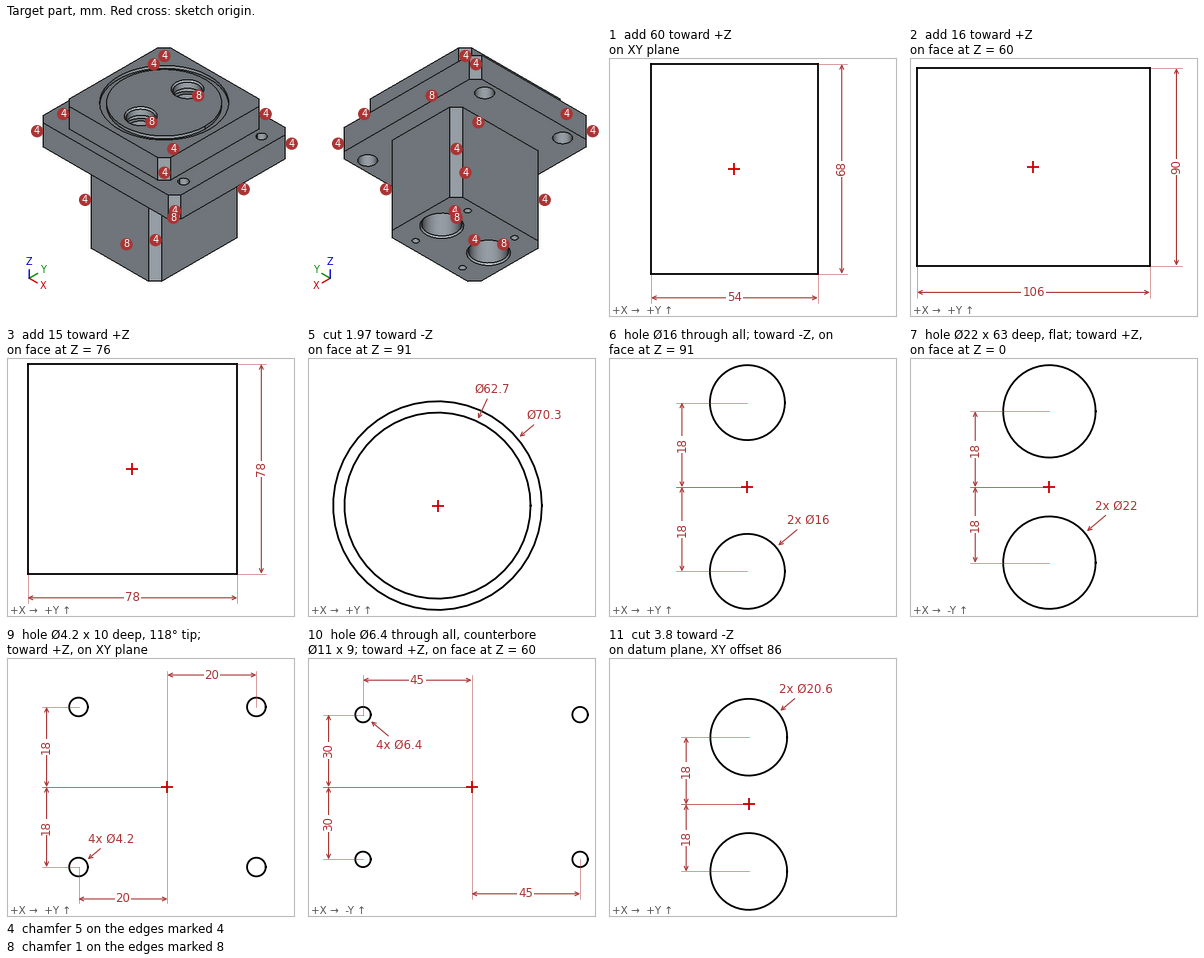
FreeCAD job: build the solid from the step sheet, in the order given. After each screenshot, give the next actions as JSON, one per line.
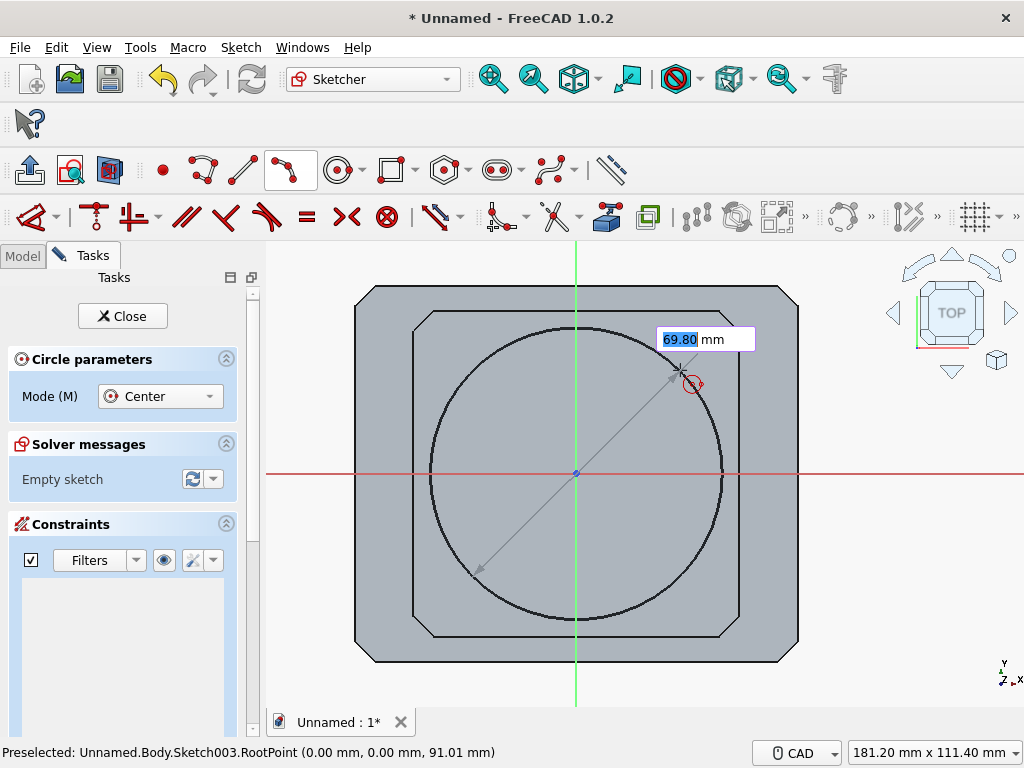
{"action": "type", "text": "70.3"}
{"action": "key", "text": "Return"}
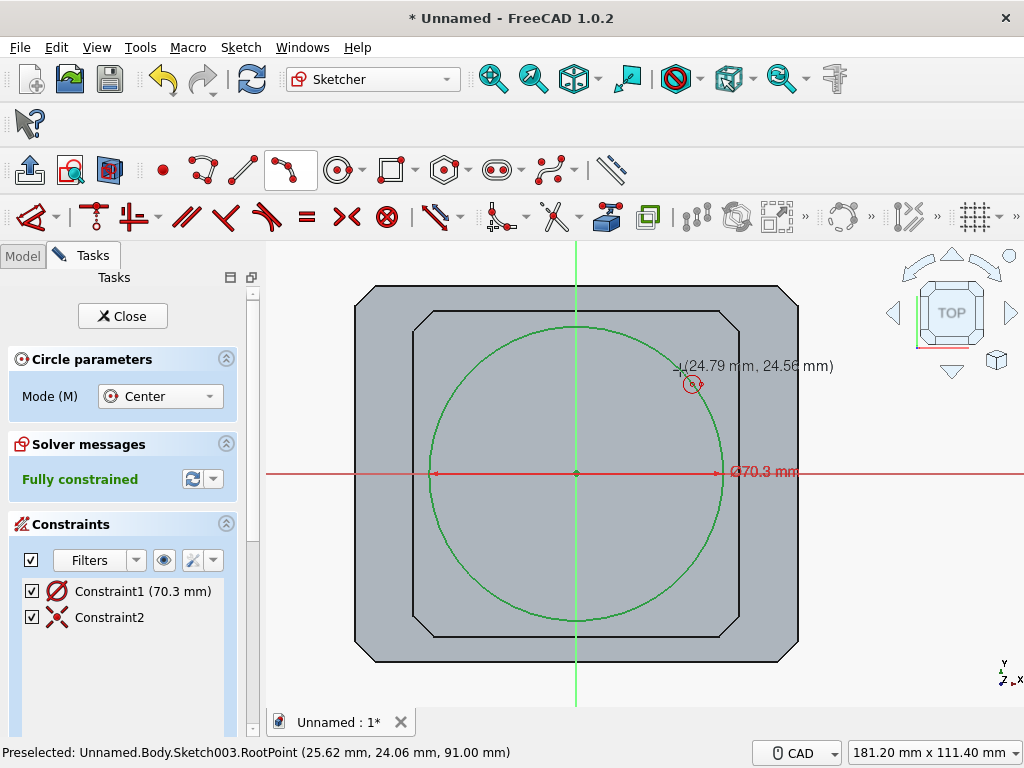
{"action": "left_click", "coordinate": [576, 474]}
{"action": "mouse_move", "coordinate": [669, 381]}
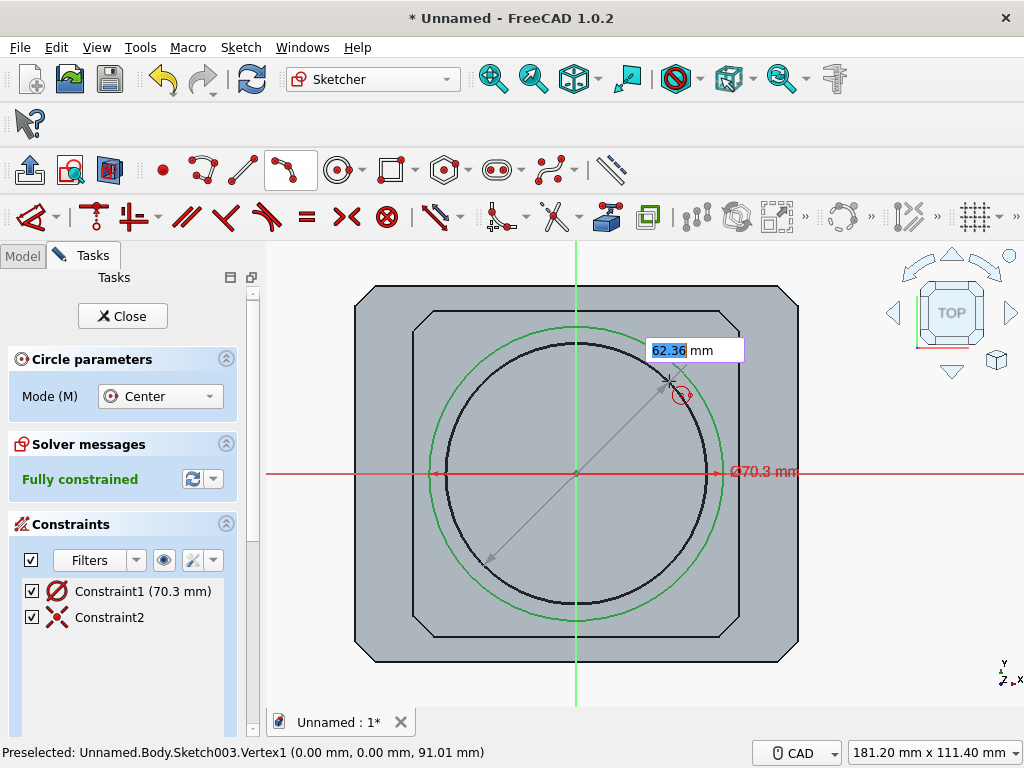
{"action": "type", "text": "62.7"}
{"action": "key", "text": "Return"}
{"action": "key", "text": "Escape"}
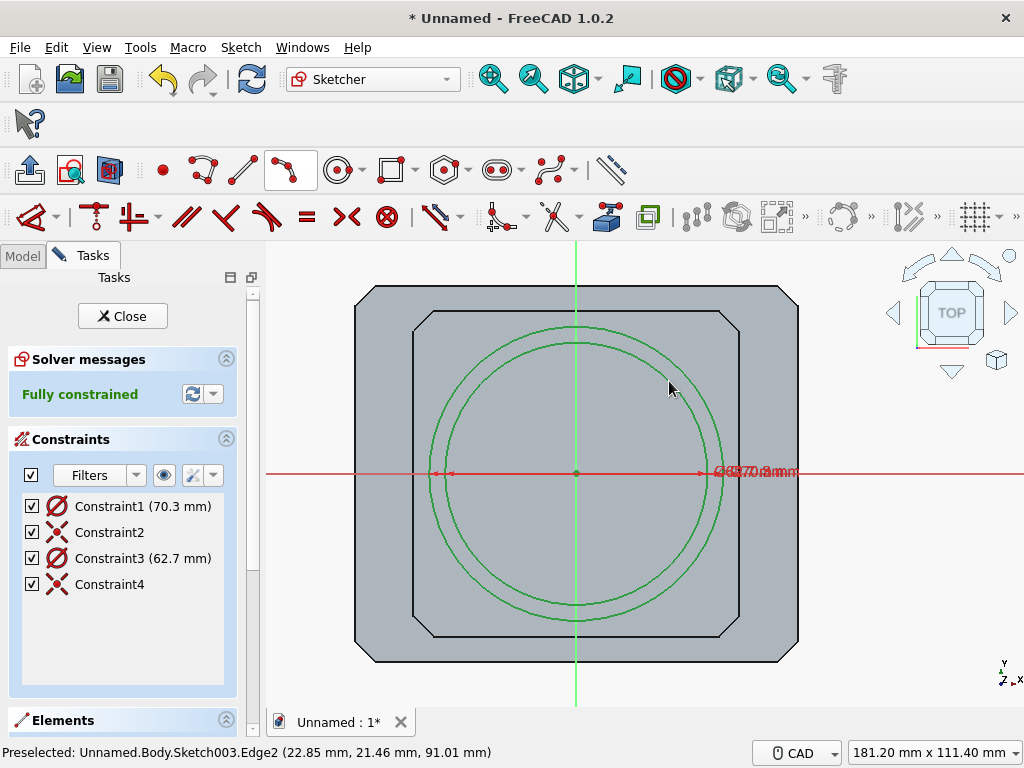
{"action": "left_click", "coordinate": [123, 316]}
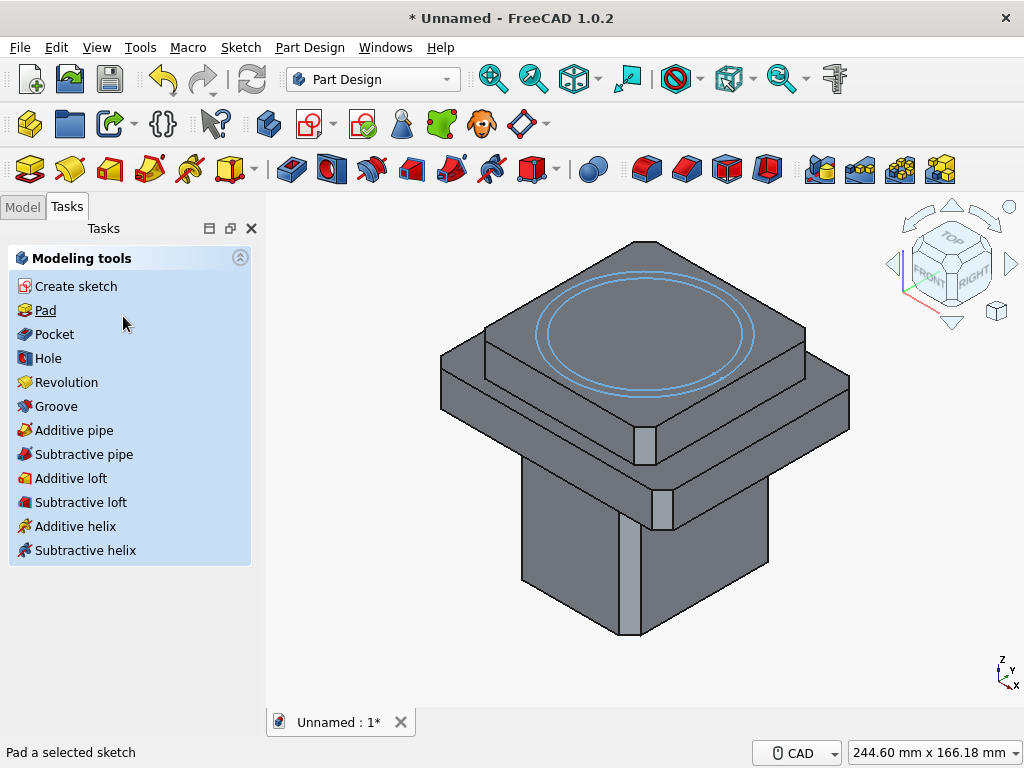
{"action": "left_click", "coordinate": [292, 170]}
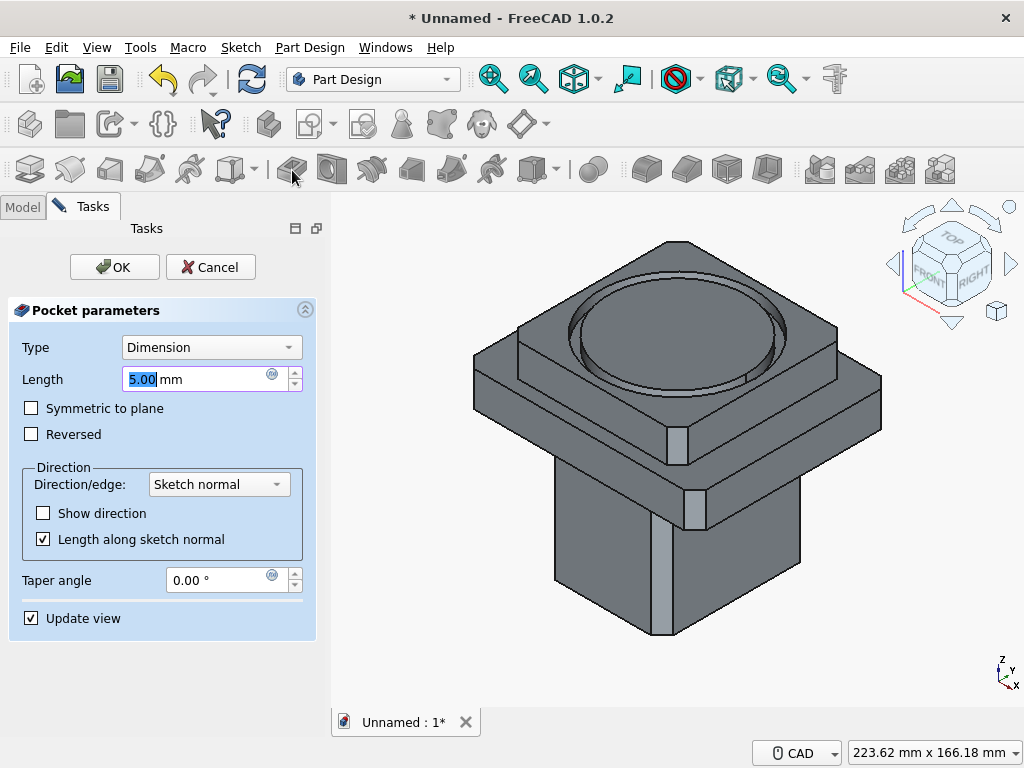
{"action": "type", "text": "1.97"}
{"action": "key", "text": "Tab"}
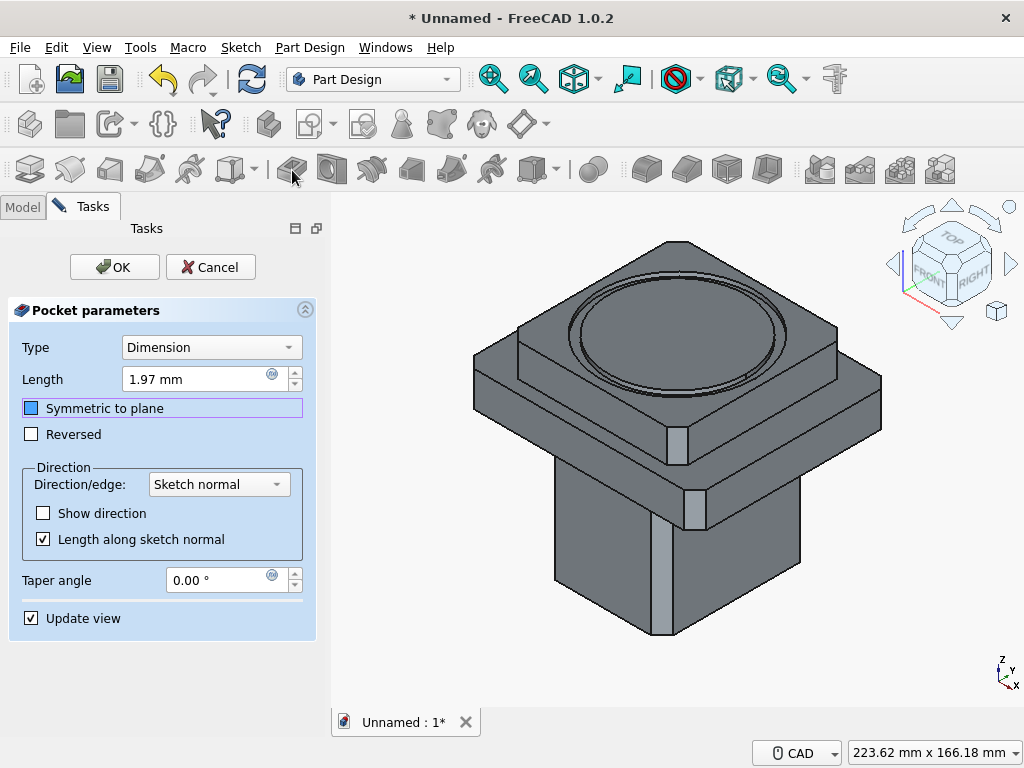
{"action": "left_click", "coordinate": [115, 267]}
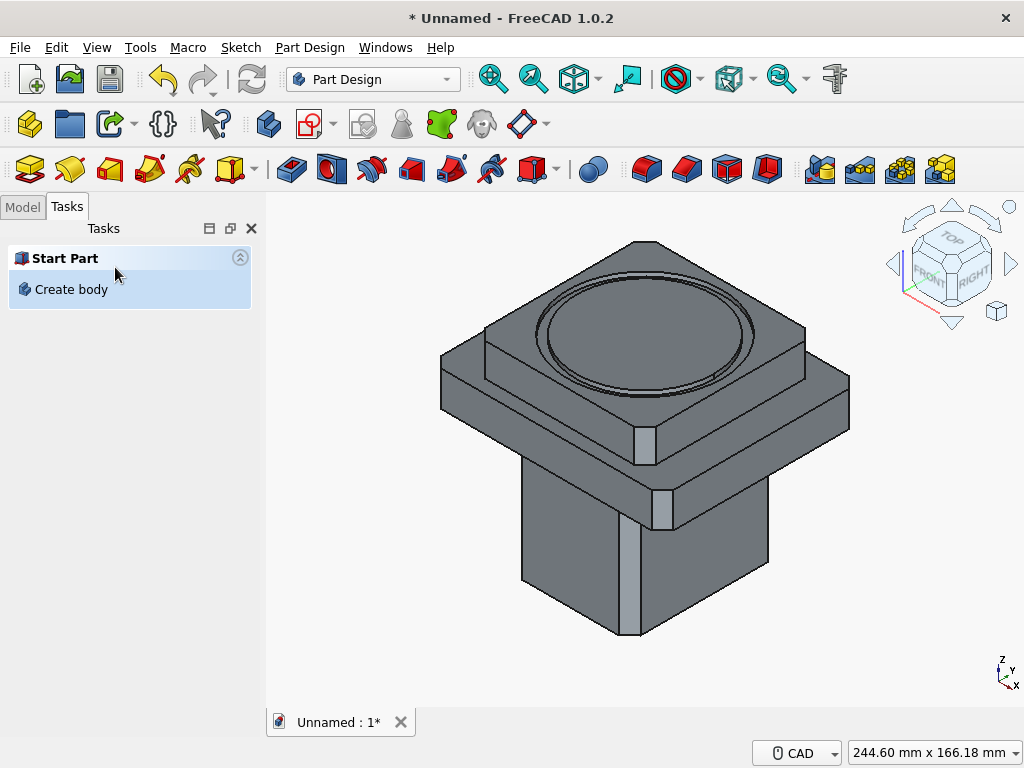
{"action": "left_click", "coordinate": [645, 333]}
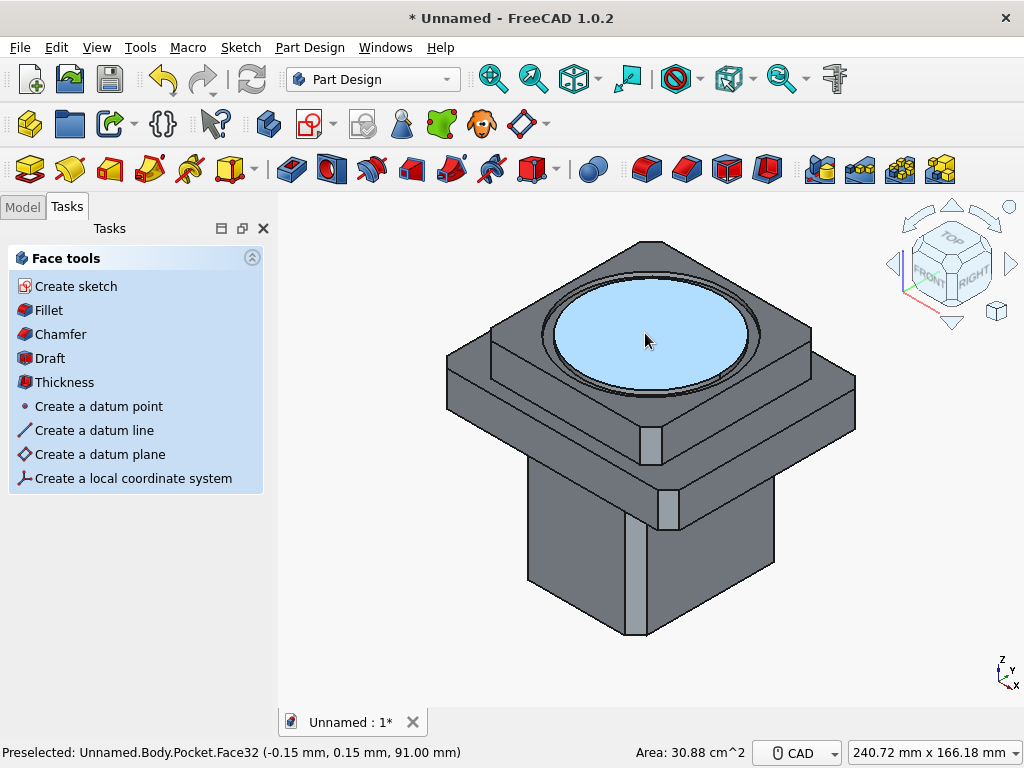
{"action": "left_click", "coordinate": [310, 124]}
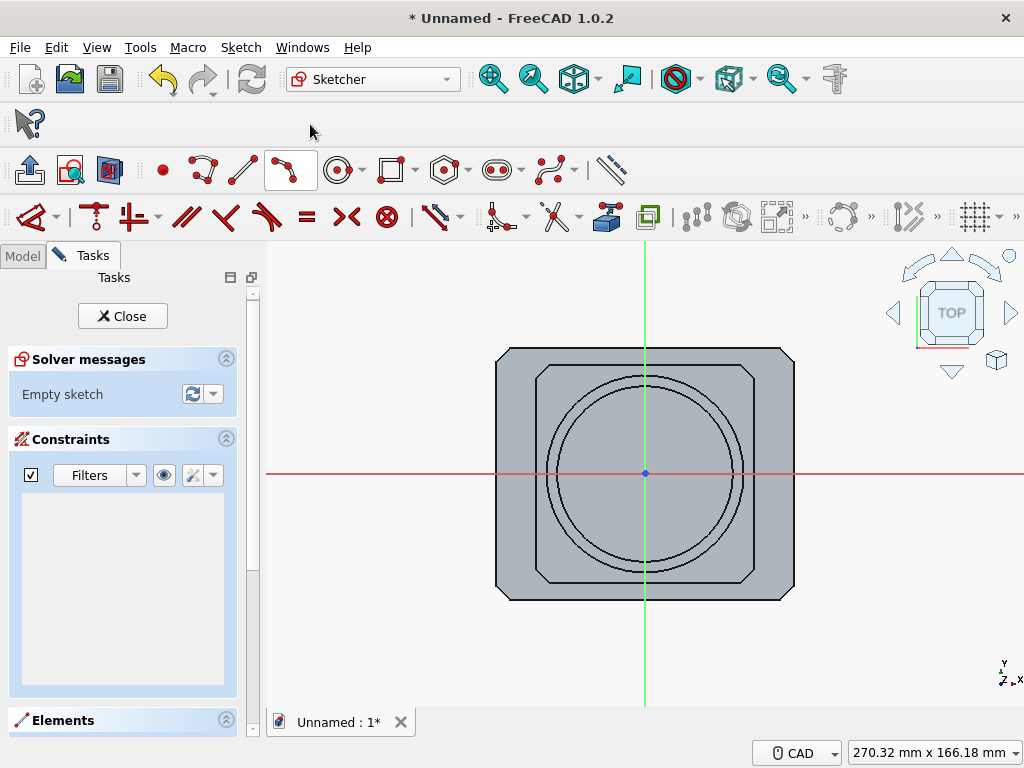
{"action": "scroll", "coordinate": [728, 474], "scroll_direction": "up", "scroll_amount": 3}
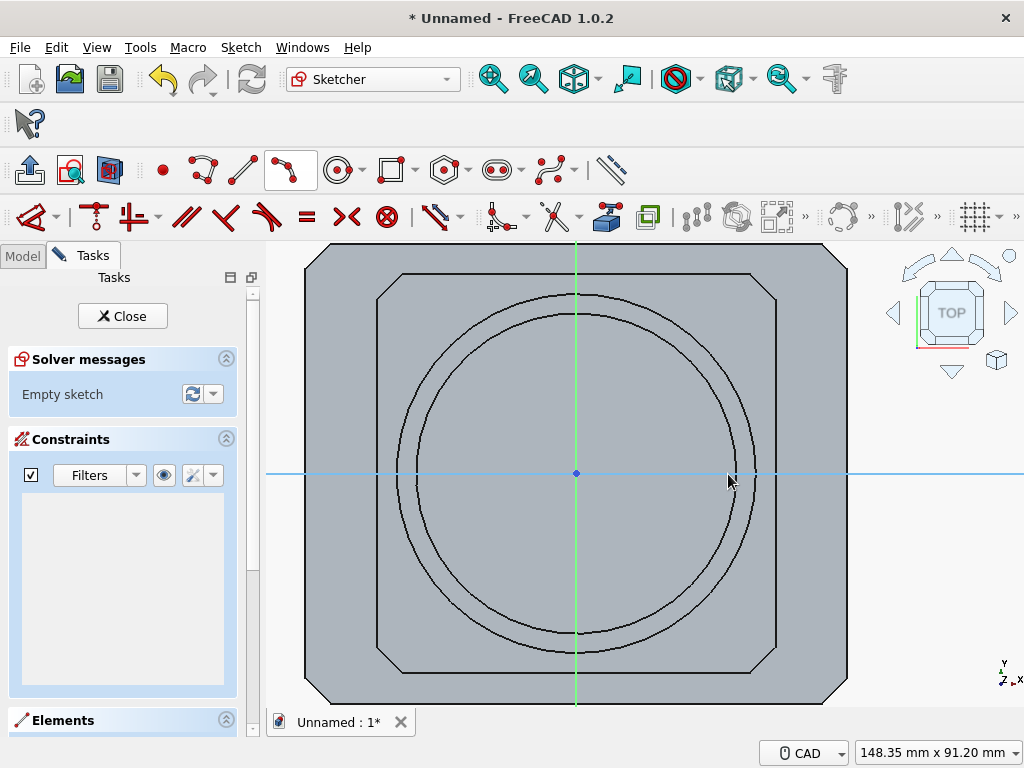
{"action": "left_click", "coordinate": [338, 170]}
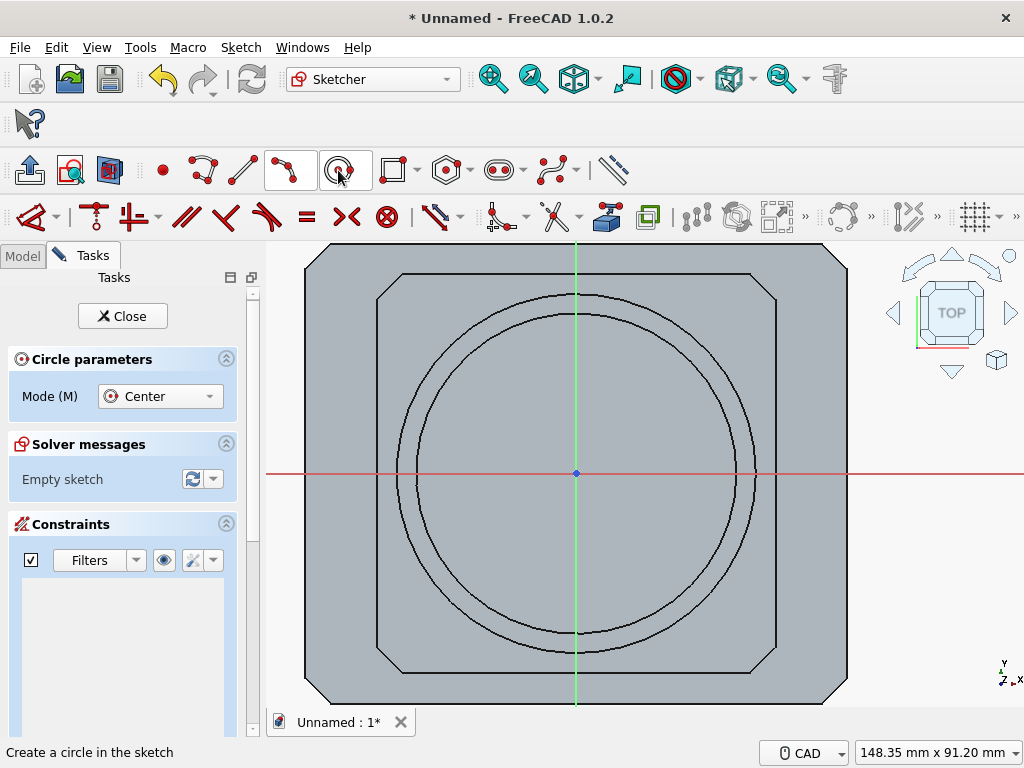
{"action": "left_click", "coordinate": [576, 566]}
{"action": "mouse_move", "coordinate": [605, 537]}